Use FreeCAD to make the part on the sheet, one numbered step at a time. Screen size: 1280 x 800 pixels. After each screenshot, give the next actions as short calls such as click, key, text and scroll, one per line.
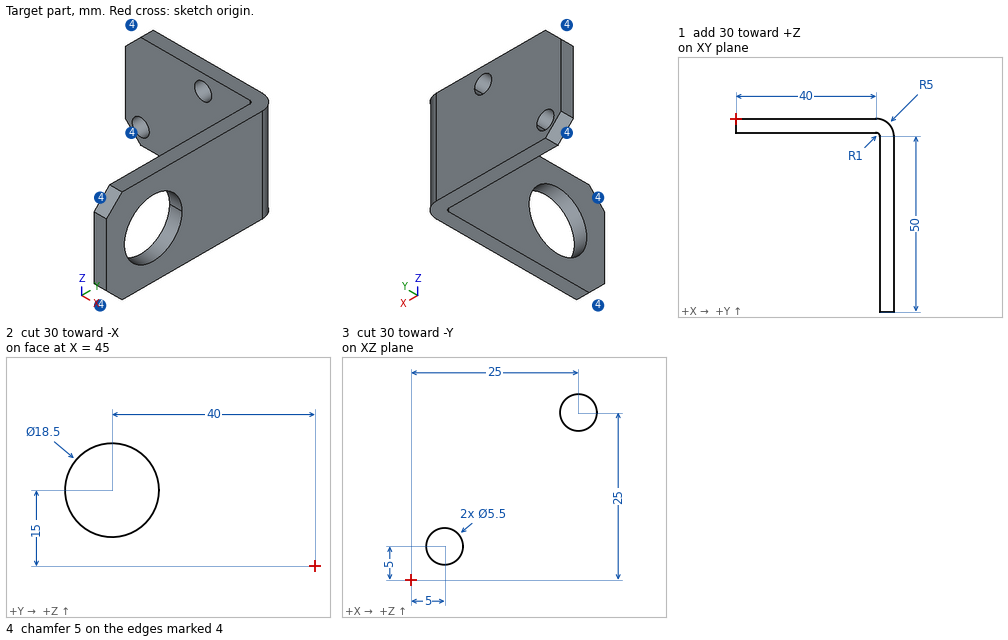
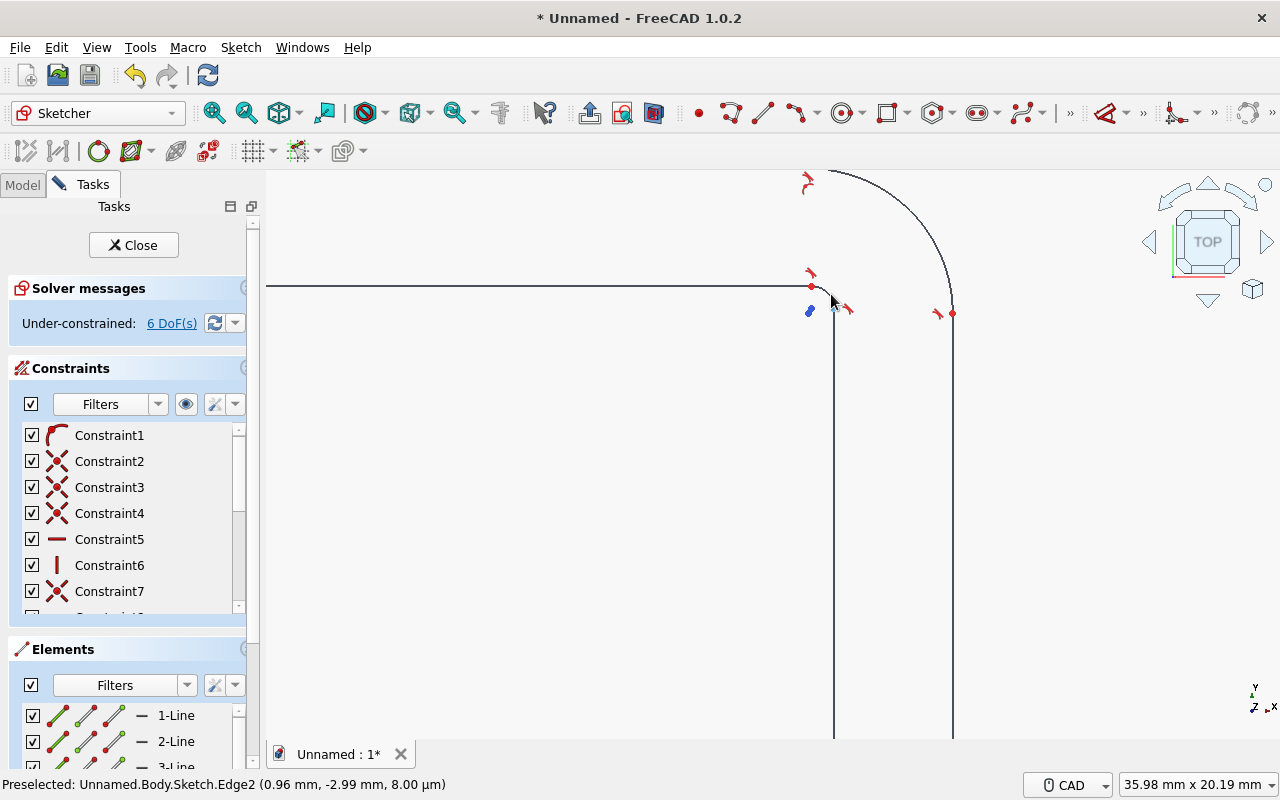
click(827, 293)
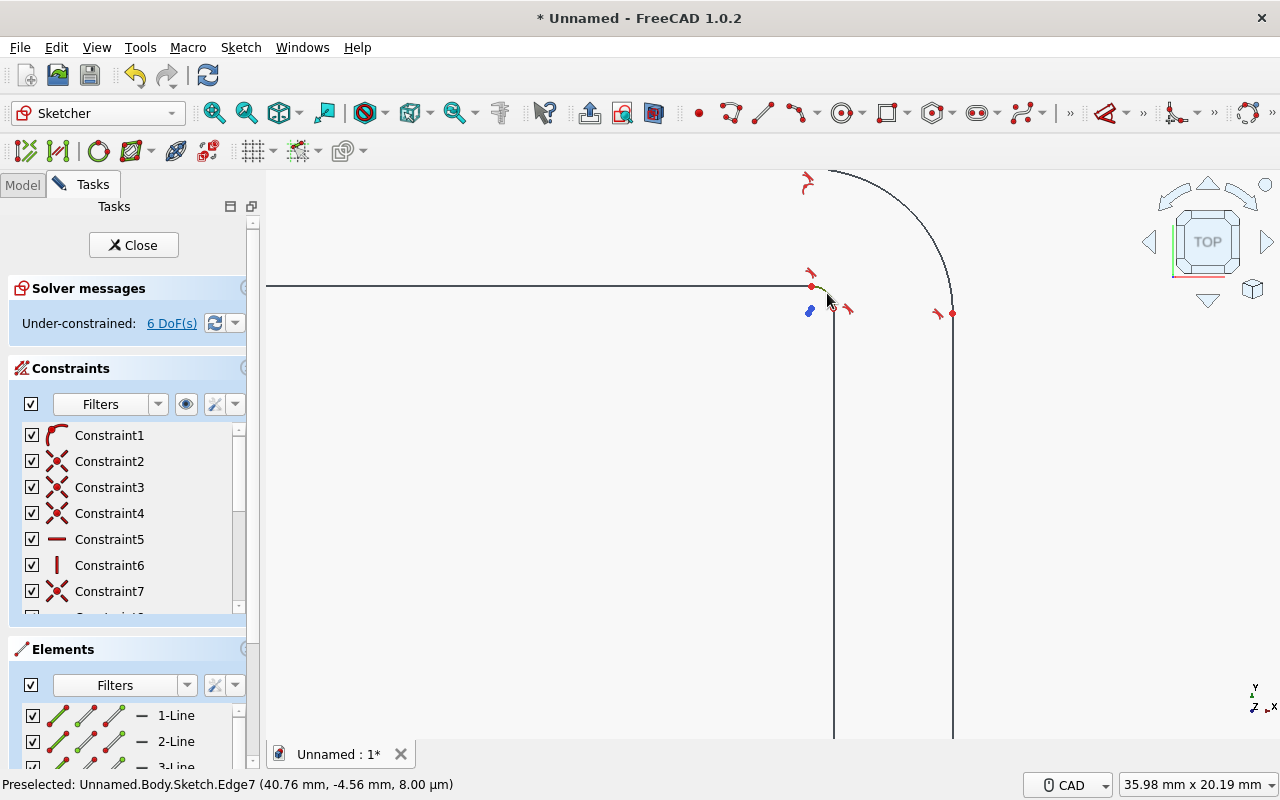
scroll(832, 294, down, 7)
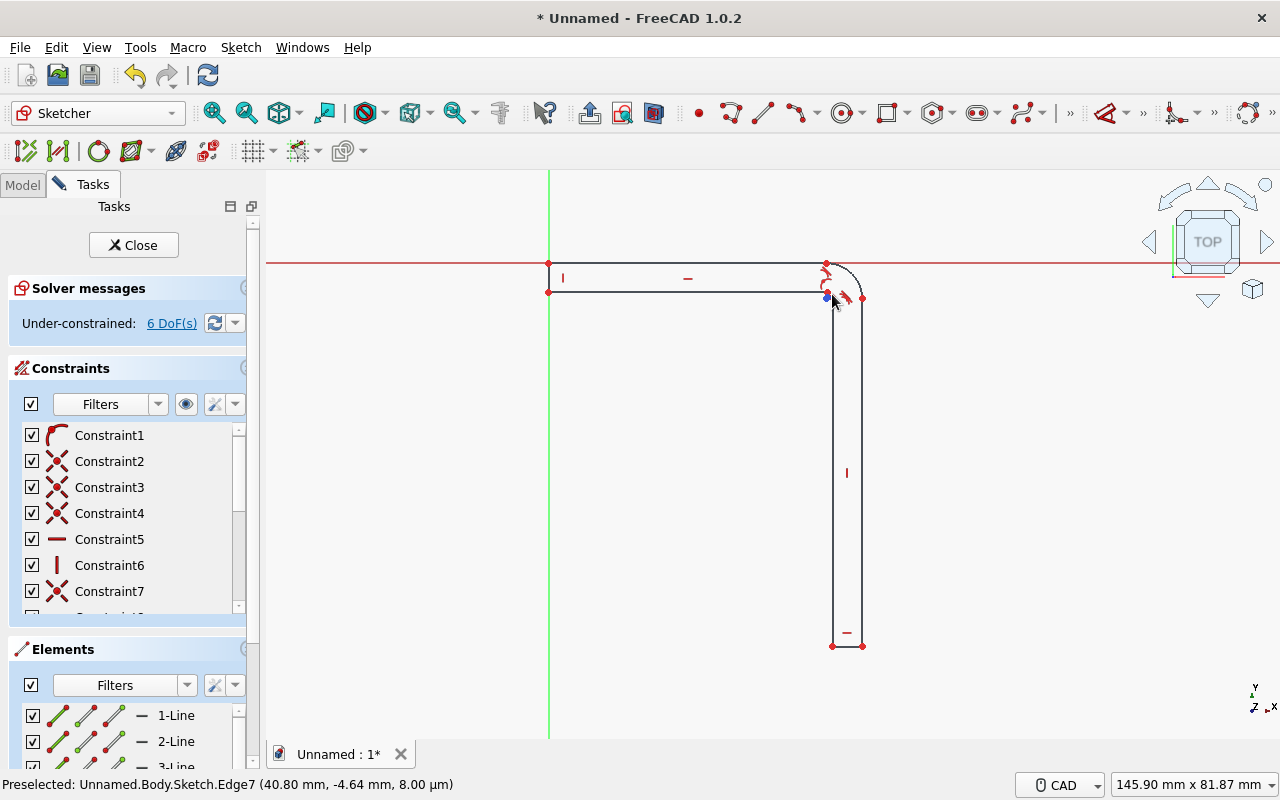
click(858, 283)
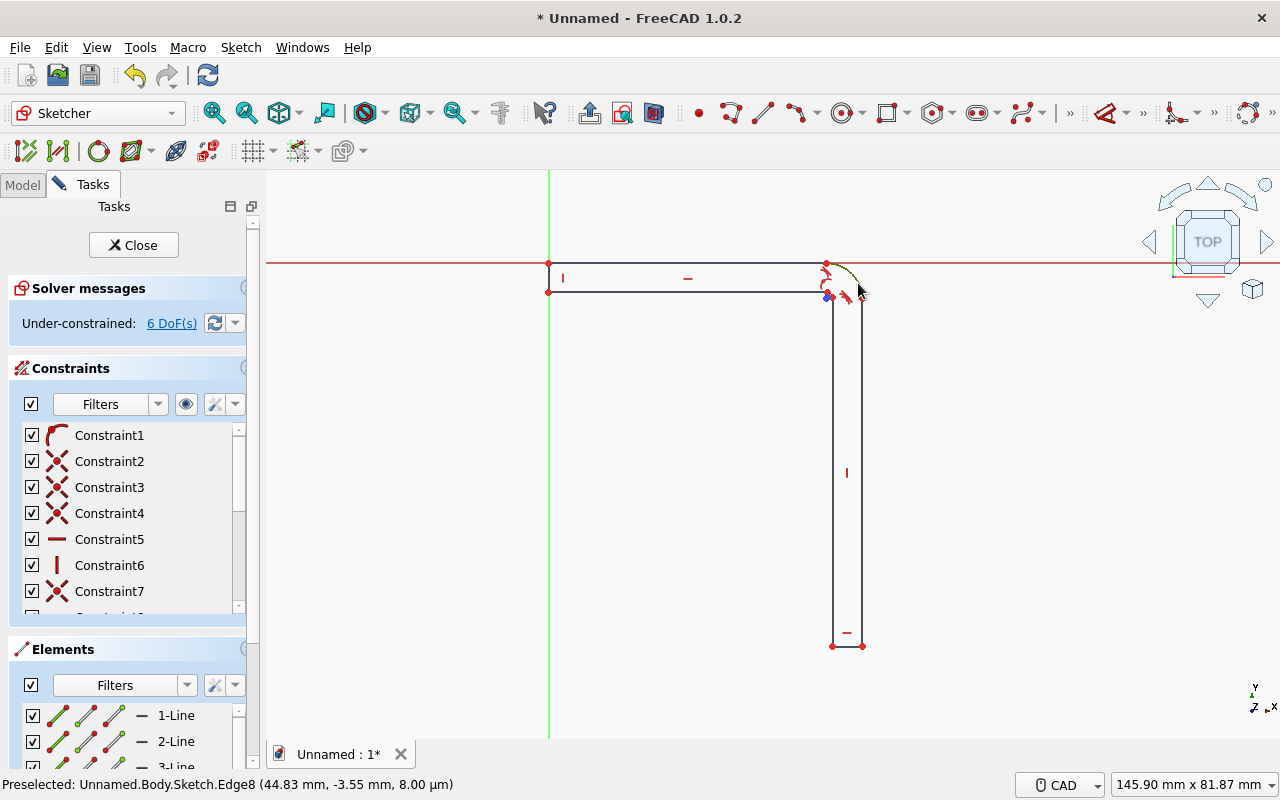
key(c)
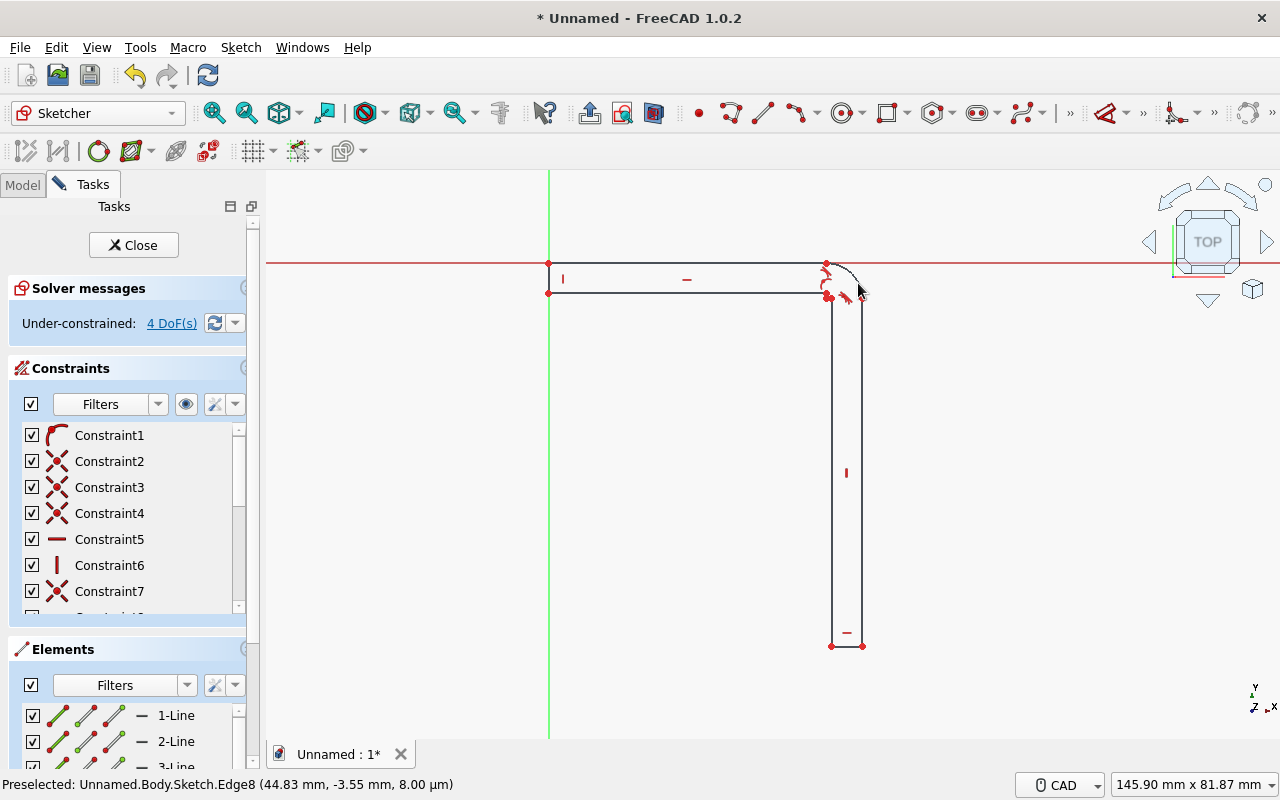
scroll(830, 295, up, 9)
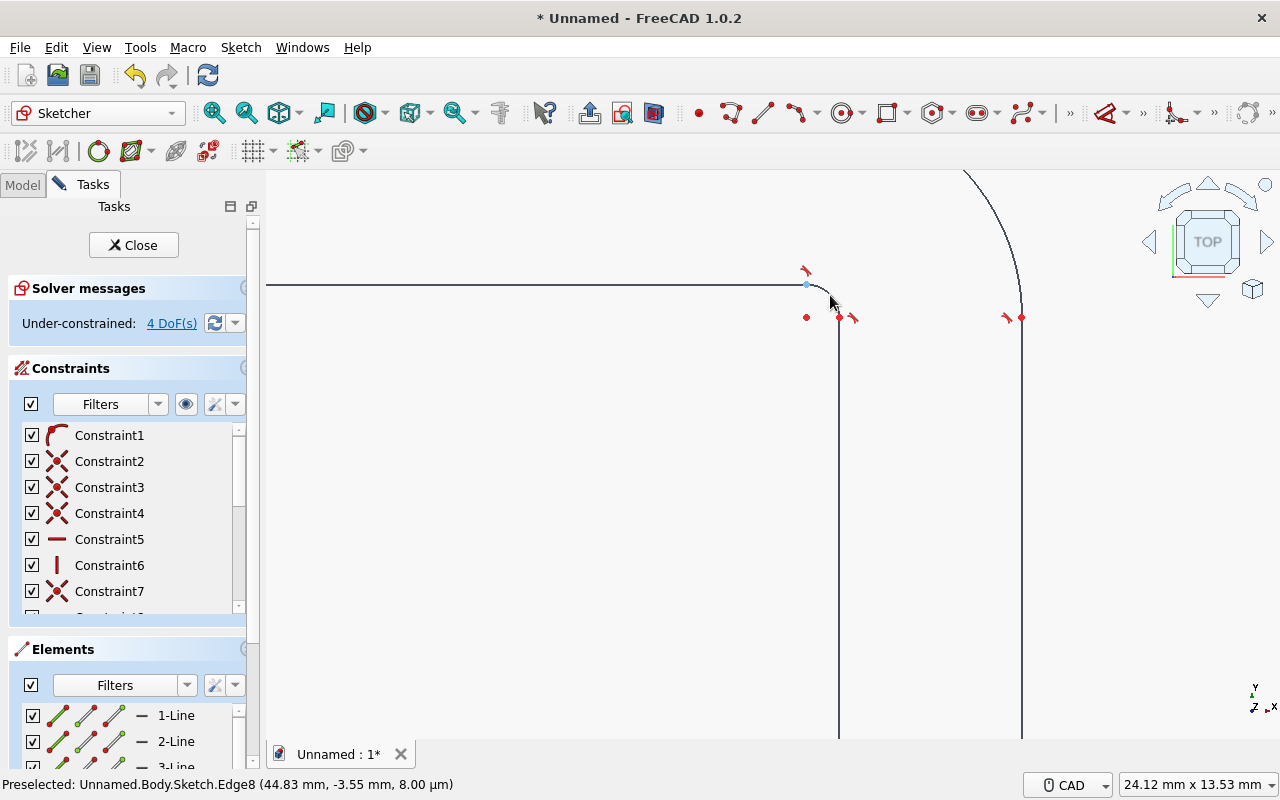
click(830, 294)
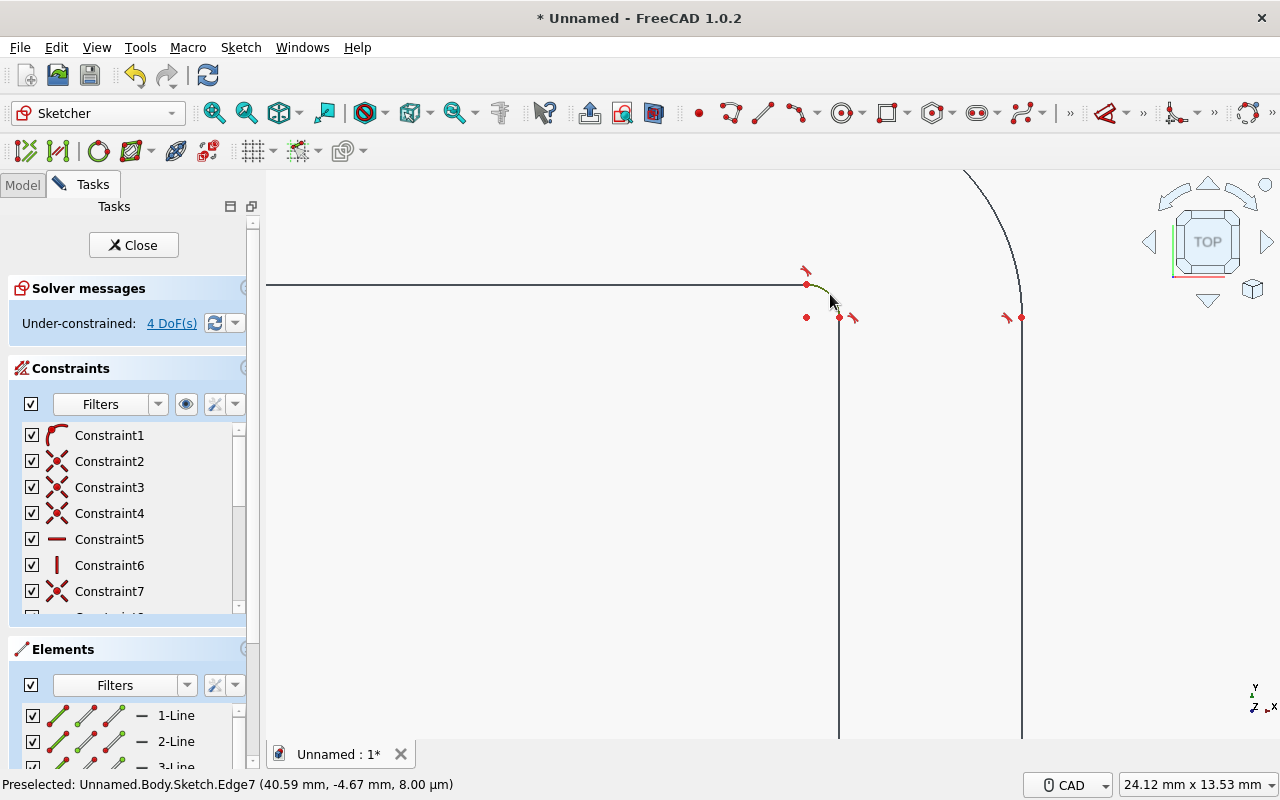
key(k)
key(r)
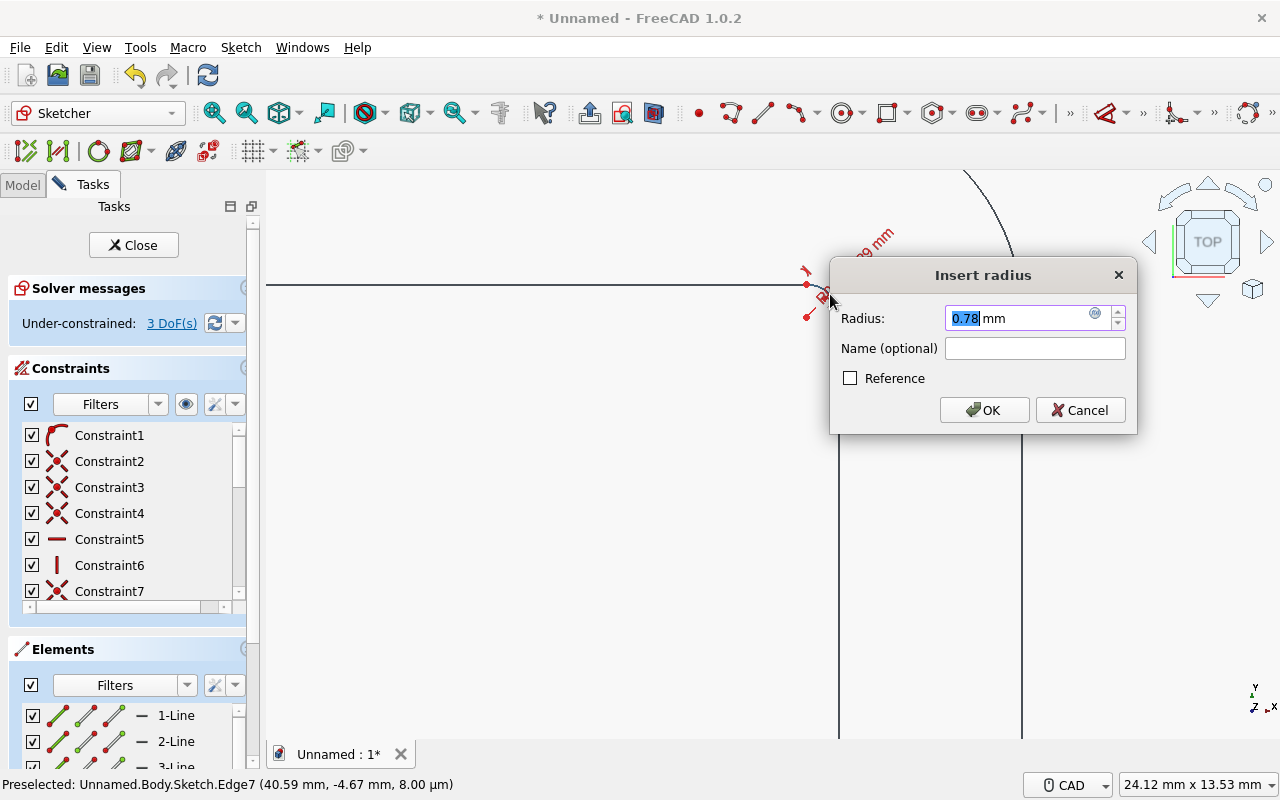
text(1)
key(Return)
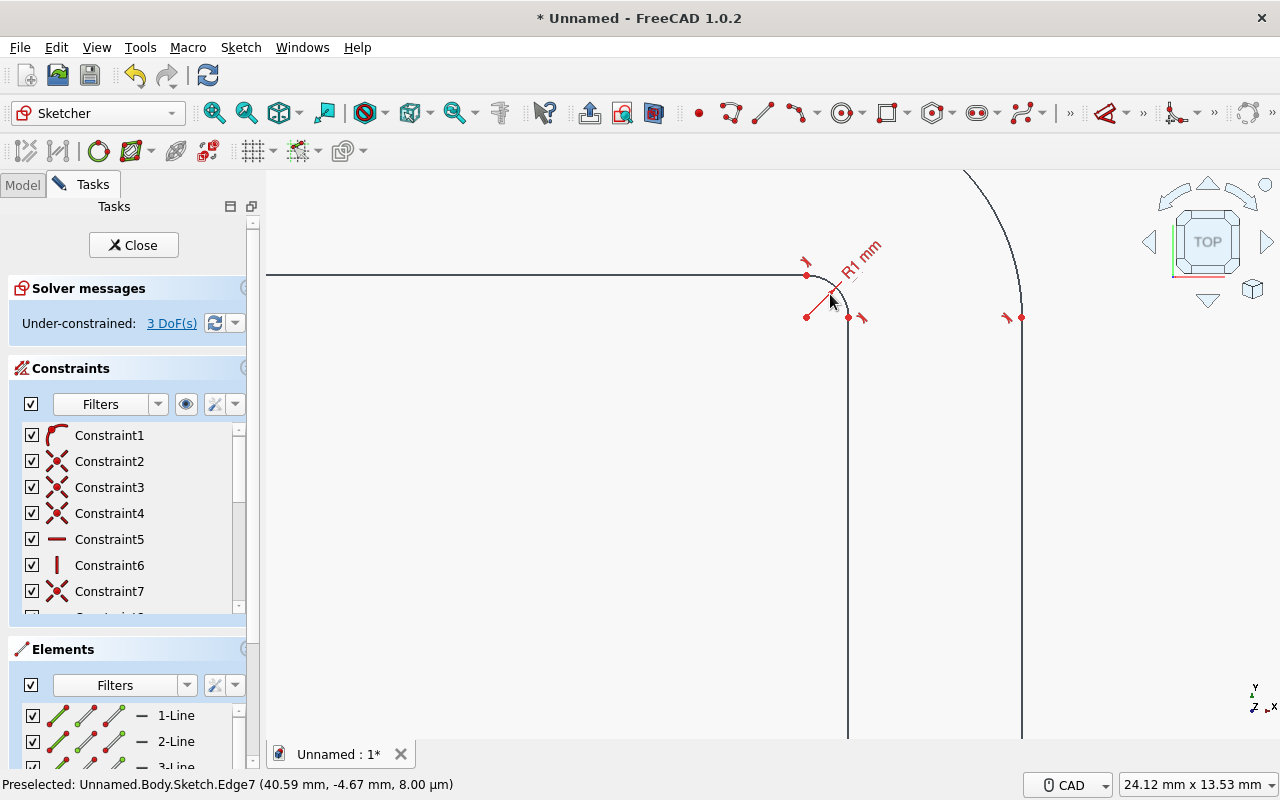
scroll(830, 295, down, 9)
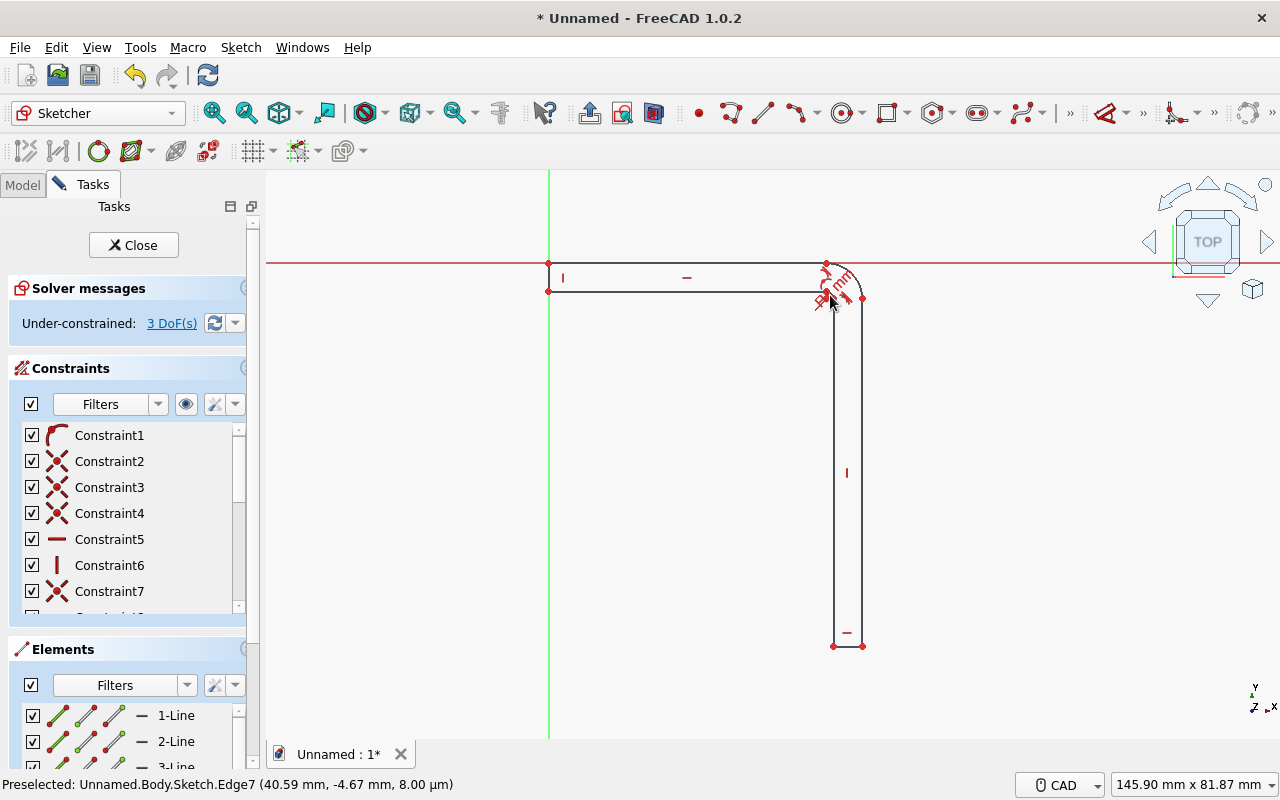
click(858, 283)